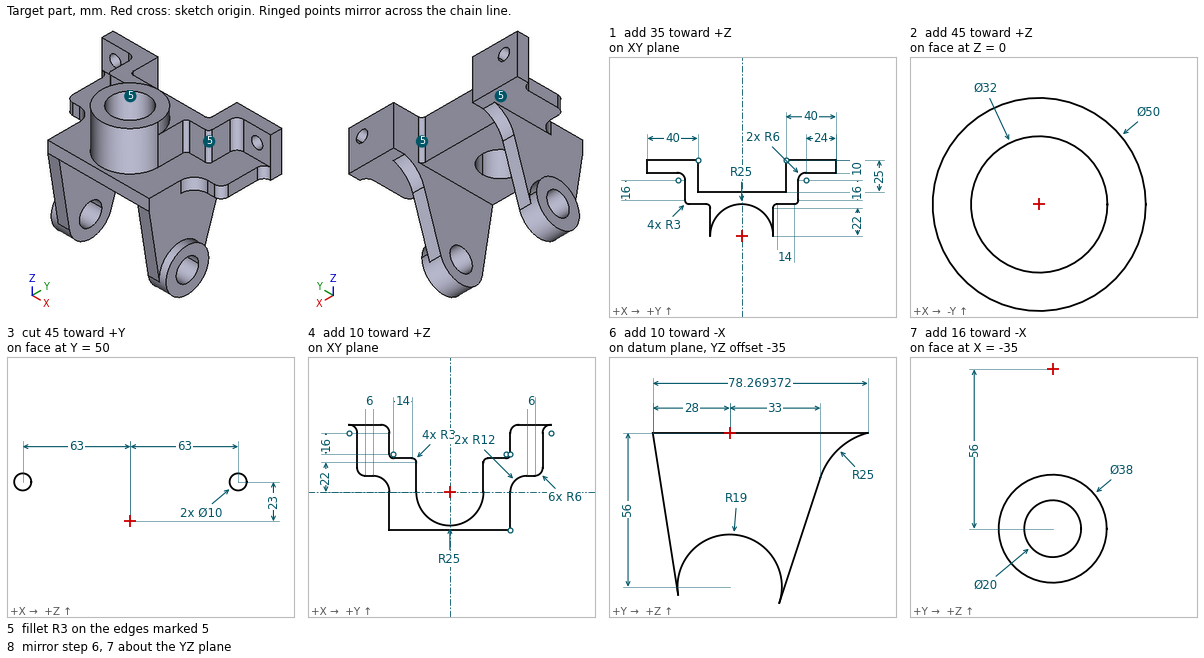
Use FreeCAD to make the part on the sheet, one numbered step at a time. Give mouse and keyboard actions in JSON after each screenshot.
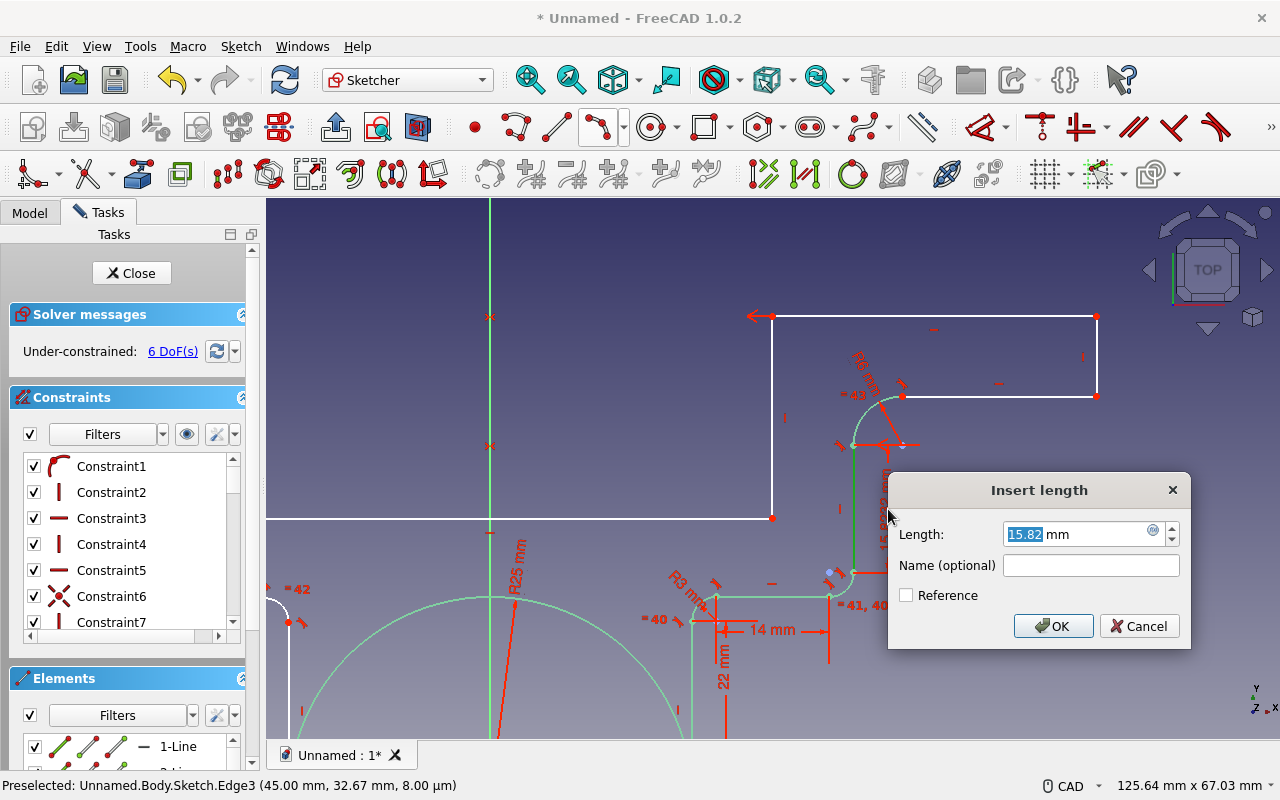
{"action": "type", "text": "16"}
{"action": "key", "text": "Return"}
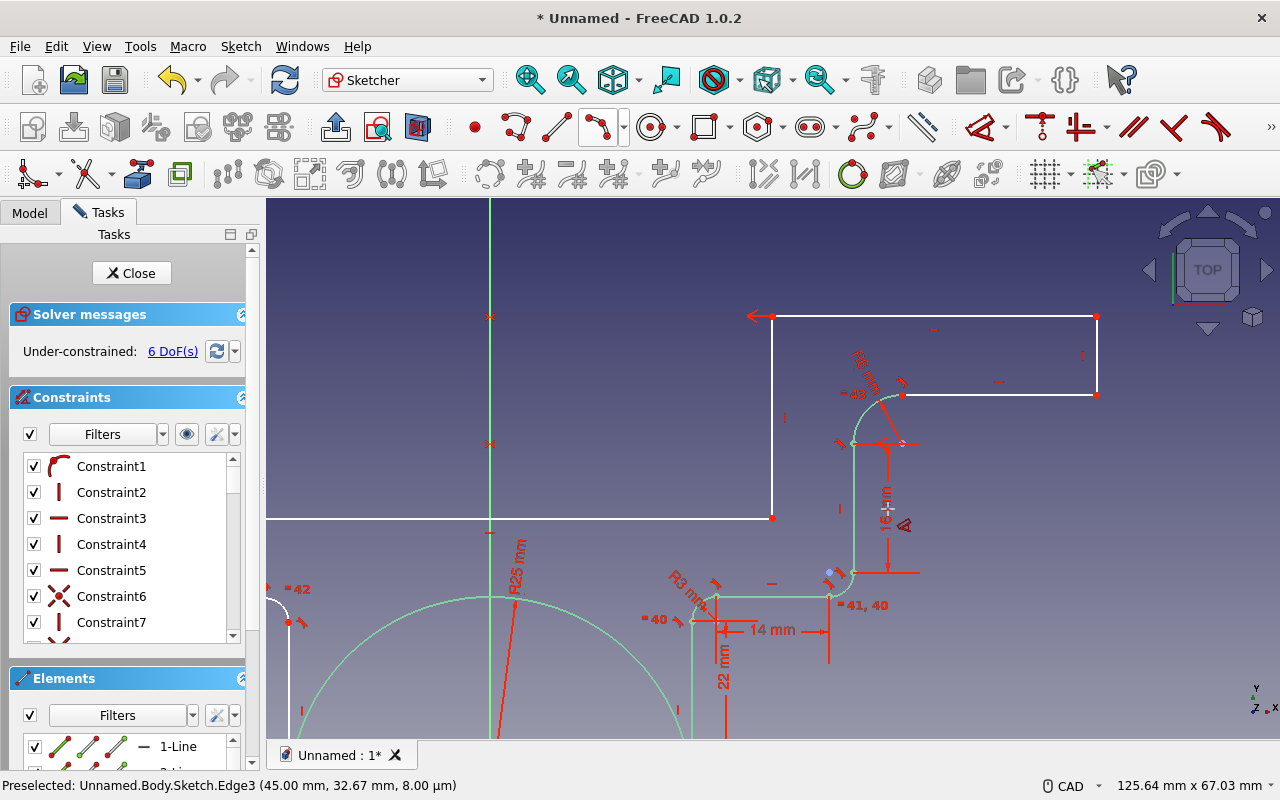
{"action": "left_click", "coordinate": [961, 395]}
{"action": "left_click", "coordinate": [1000, 361]}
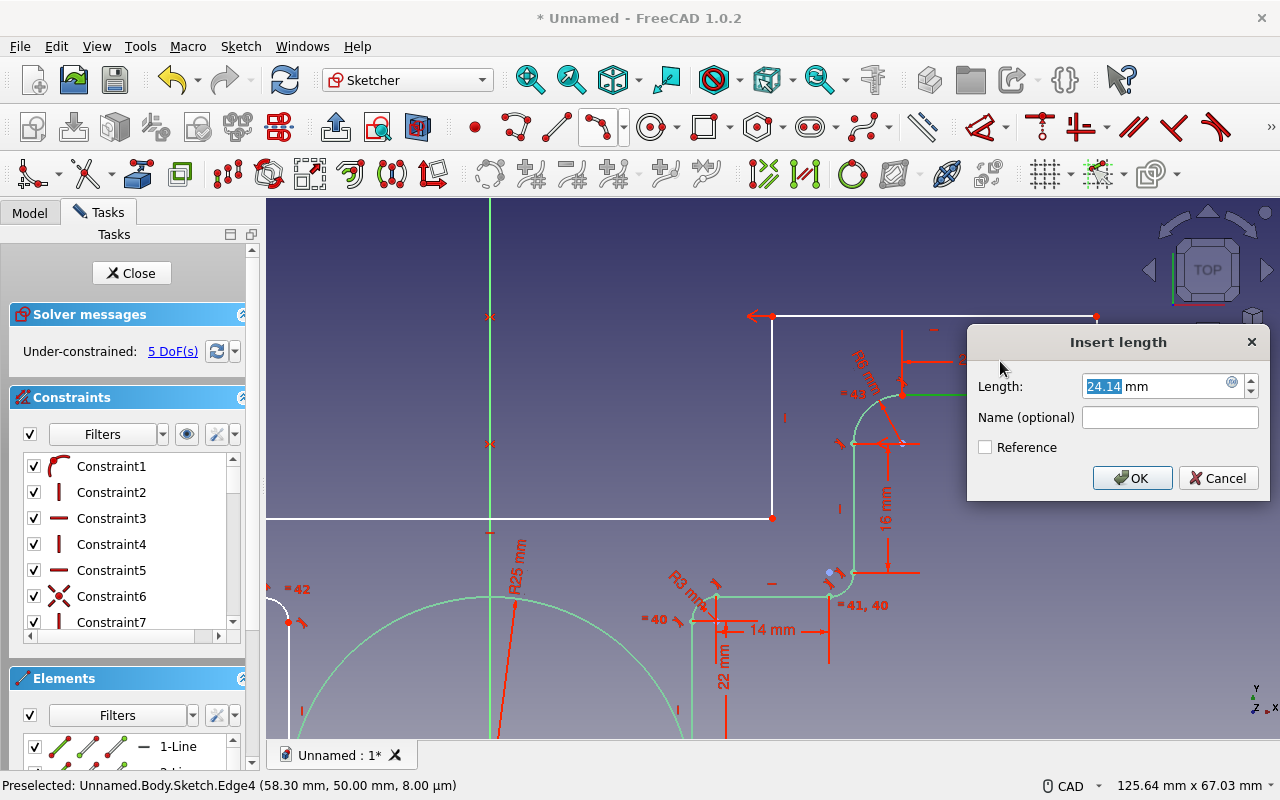
{"action": "type", "text": "24"}
{"action": "key", "text": "Return"}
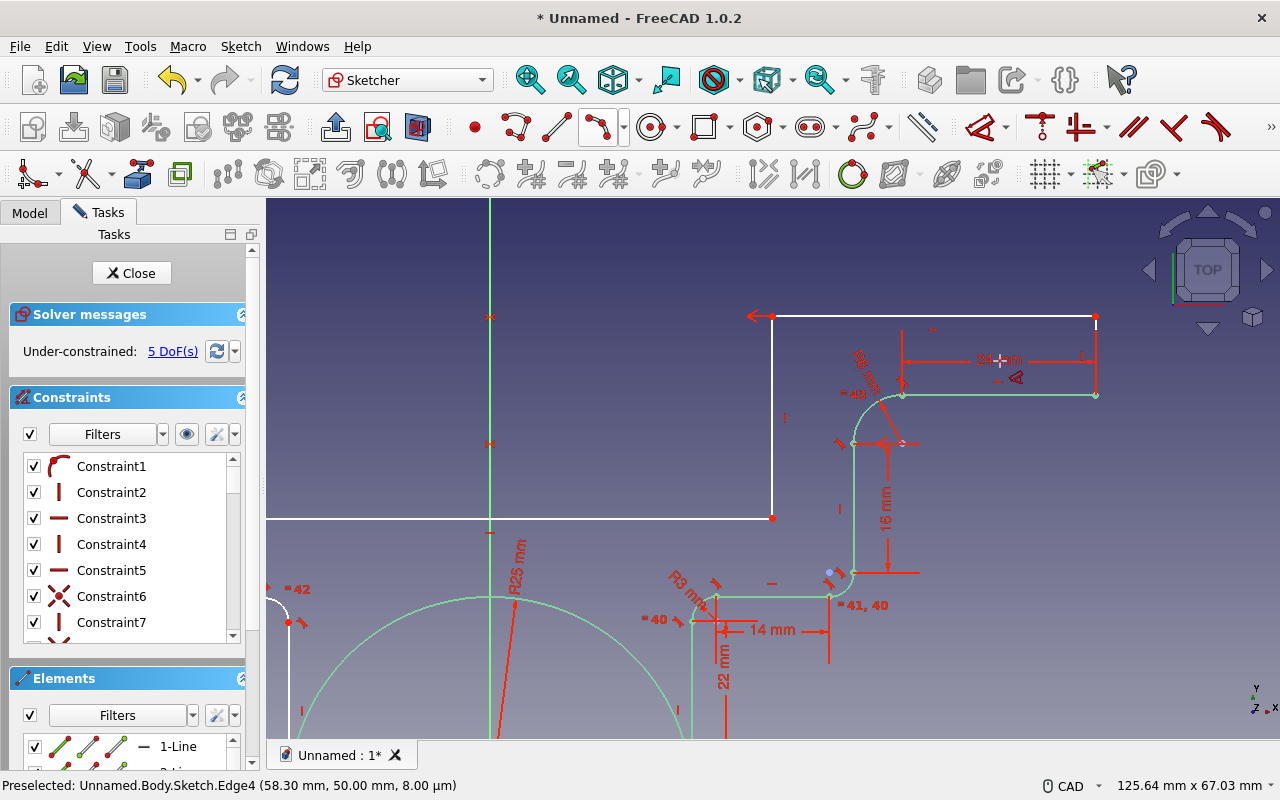
{"action": "left_click", "coordinate": [1096, 372]}
{"action": "left_click", "coordinate": [1062, 338]}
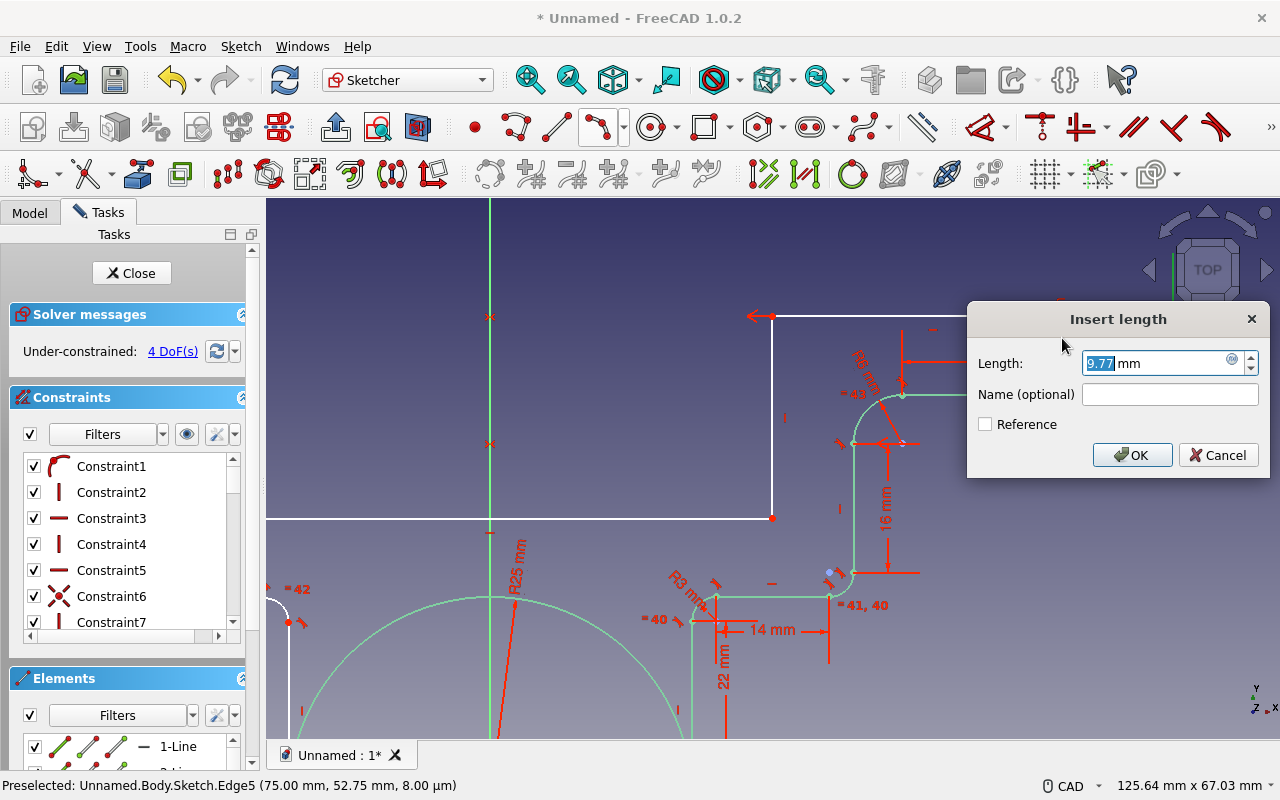
{"action": "type", "text": "10"}
{"action": "key", "text": "Return"}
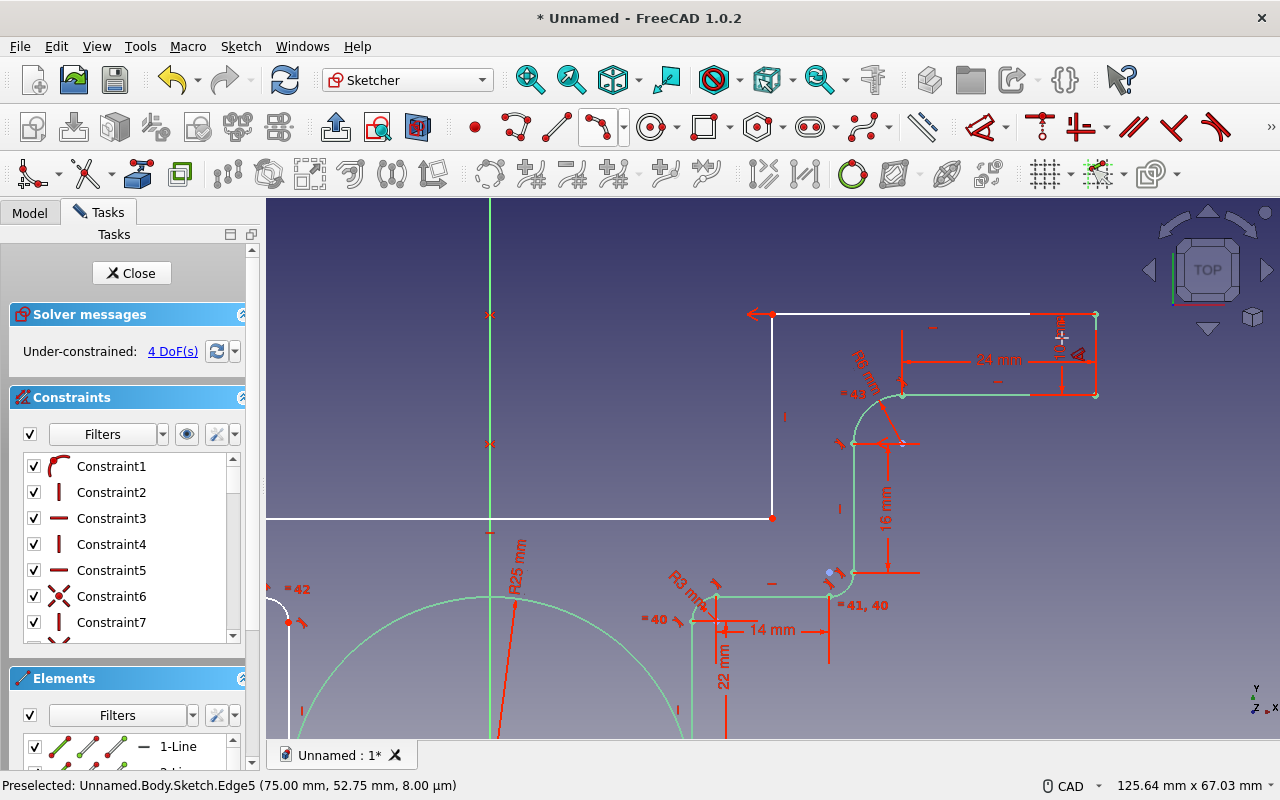
{"action": "left_click", "coordinate": [999, 314]}
{"action": "left_click", "coordinate": [934, 280]}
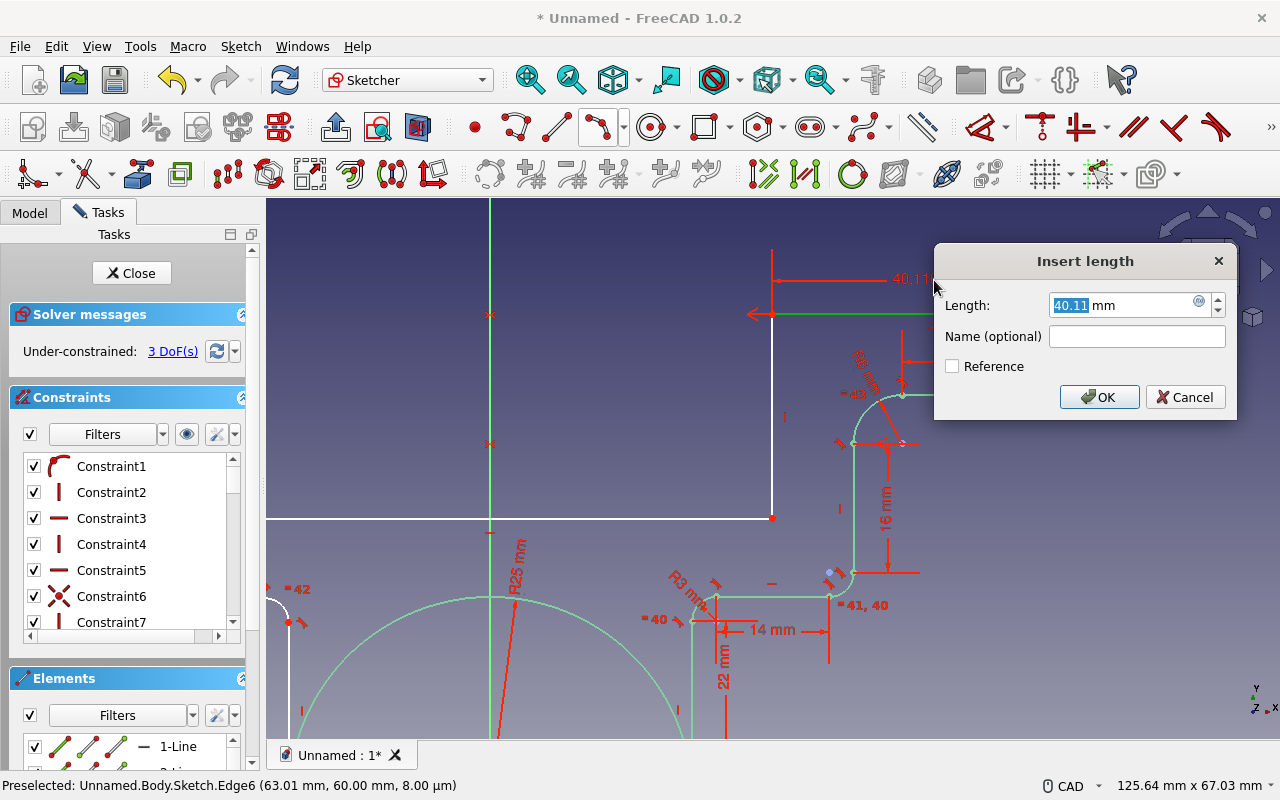
{"action": "type", "text": "40"}
{"action": "key", "text": "Return"}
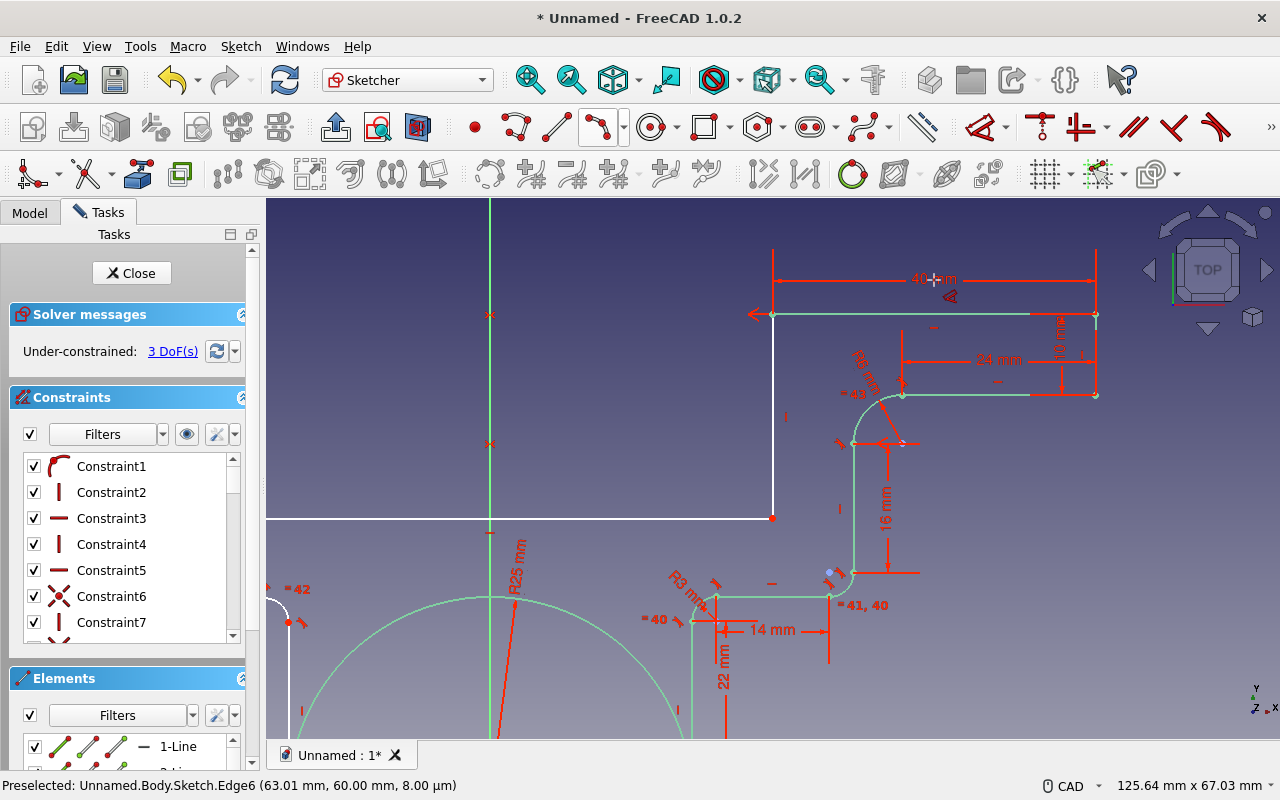
{"action": "left_click", "coordinate": [773, 376]}
{"action": "left_click", "coordinate": [807, 417]}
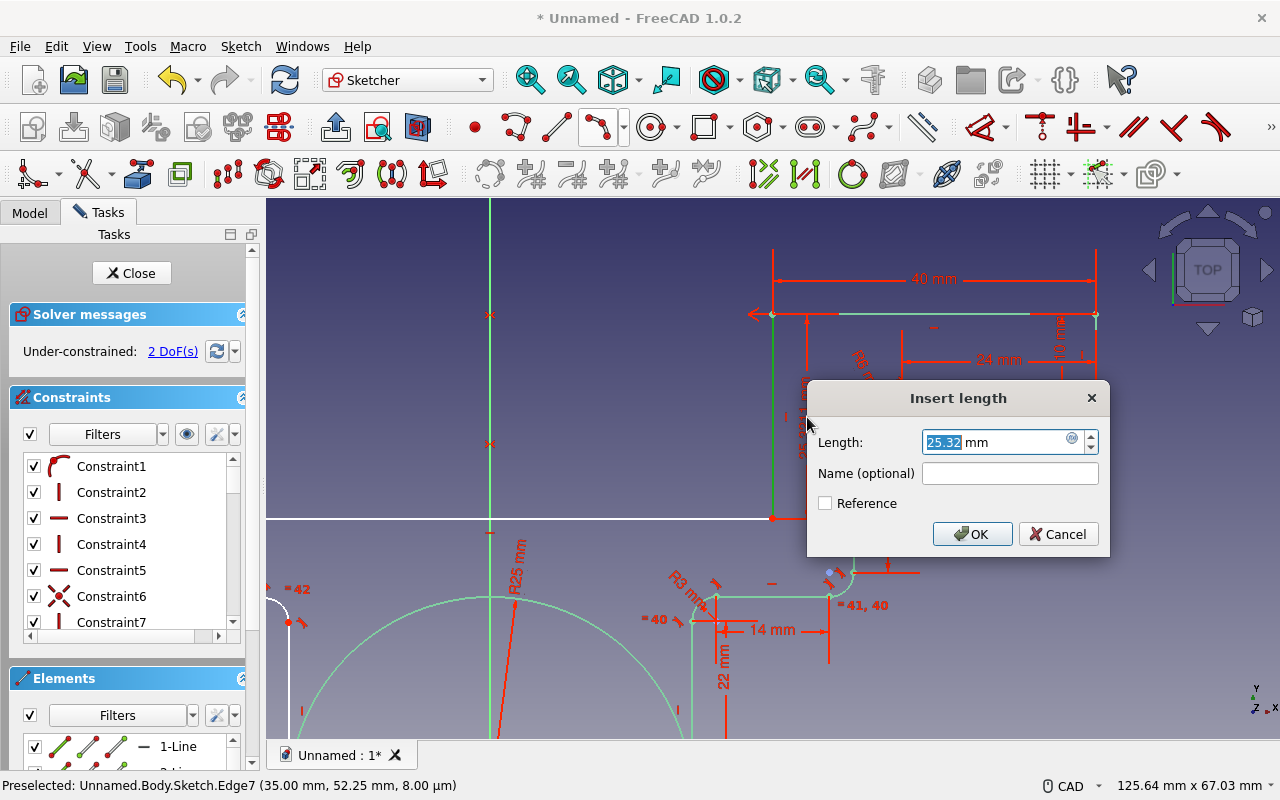
{"action": "type", "text": "25"}
{"action": "key", "text": "Return"}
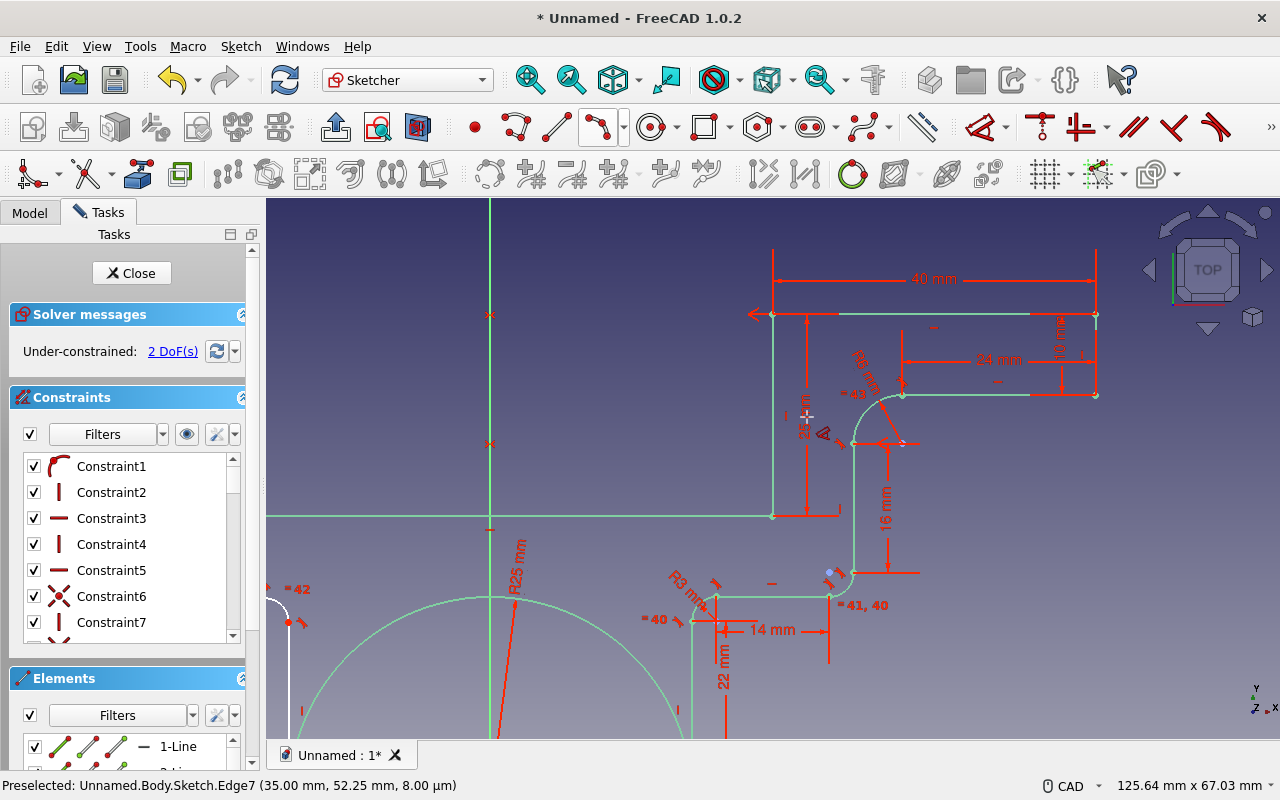
{"action": "scroll", "coordinate": [879, 397], "scroll_direction": "down", "scroll_amount": 4}